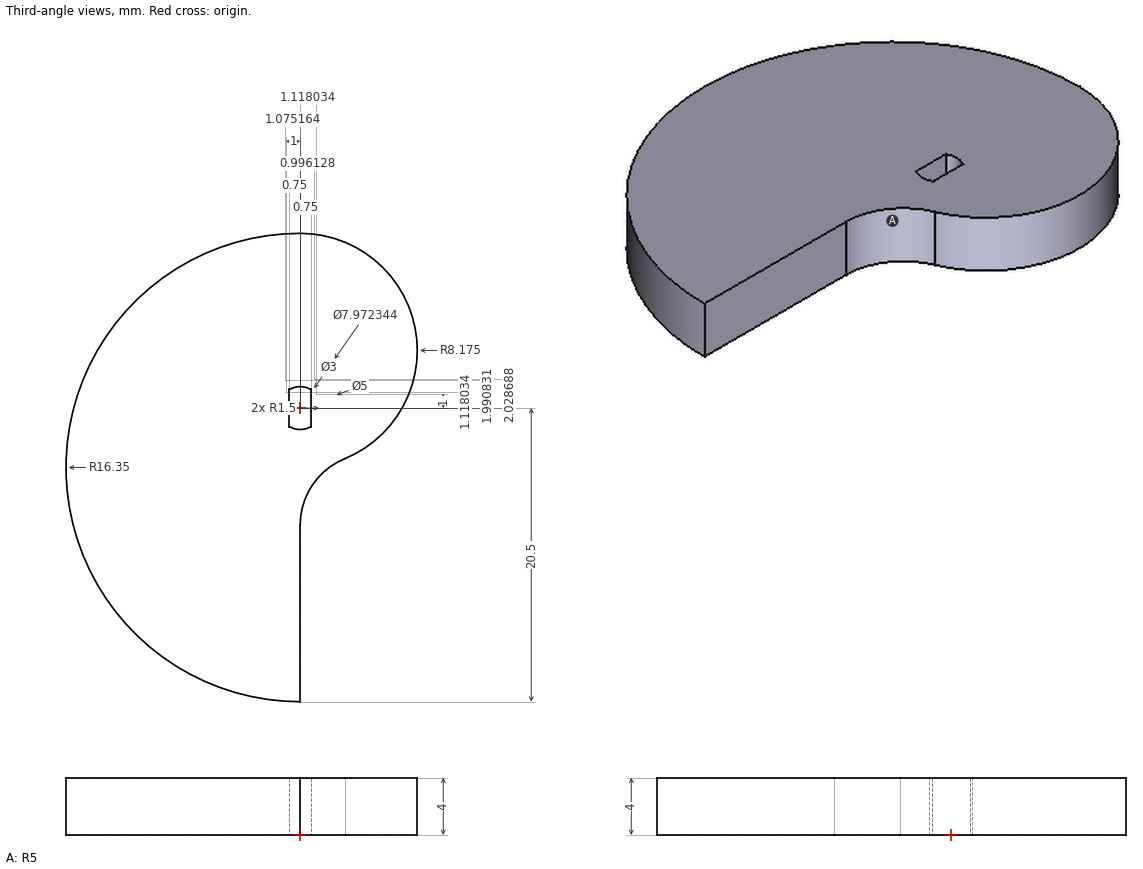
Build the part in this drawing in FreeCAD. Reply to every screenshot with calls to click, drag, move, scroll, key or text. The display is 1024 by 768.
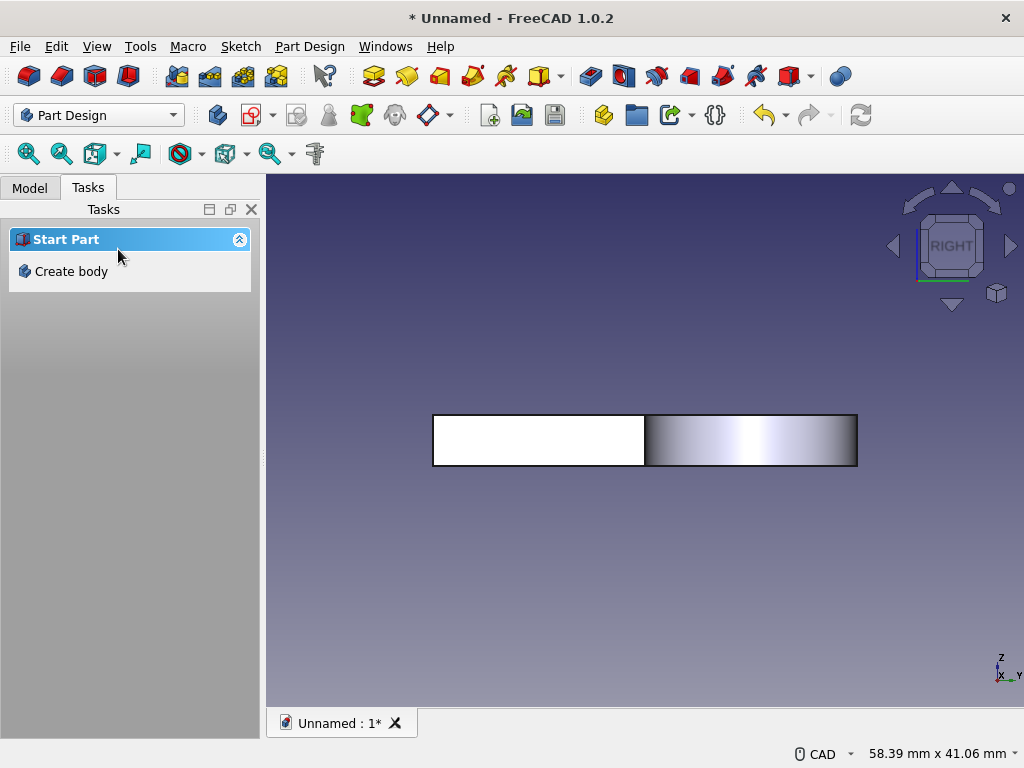
key(5)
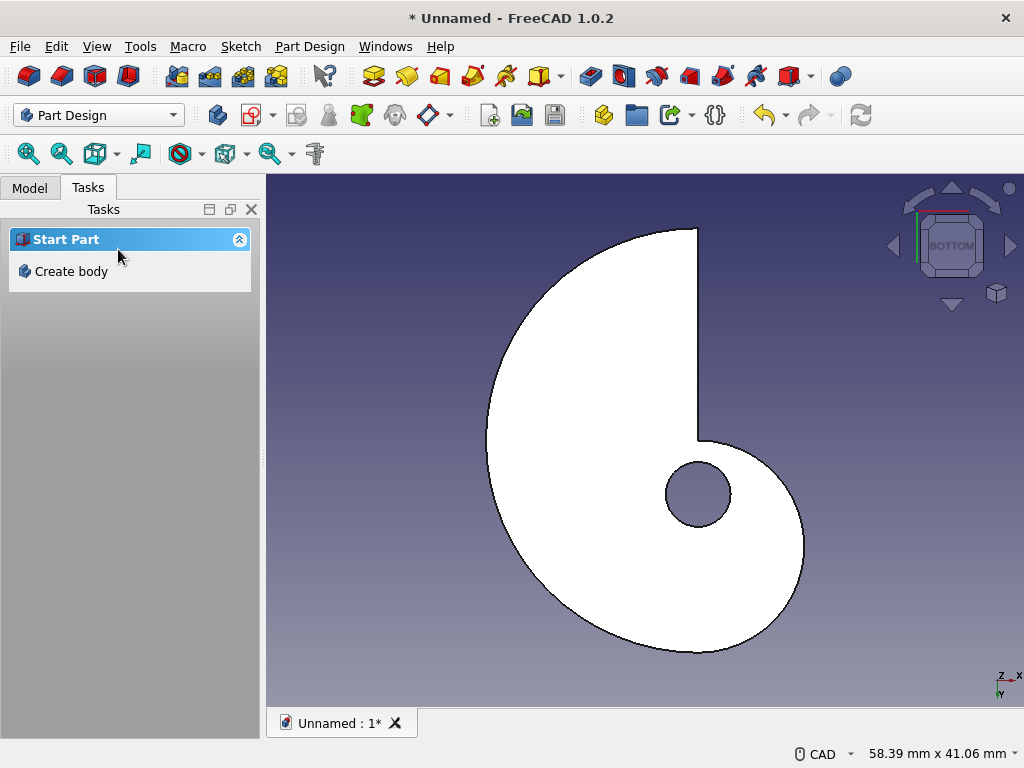
key(4)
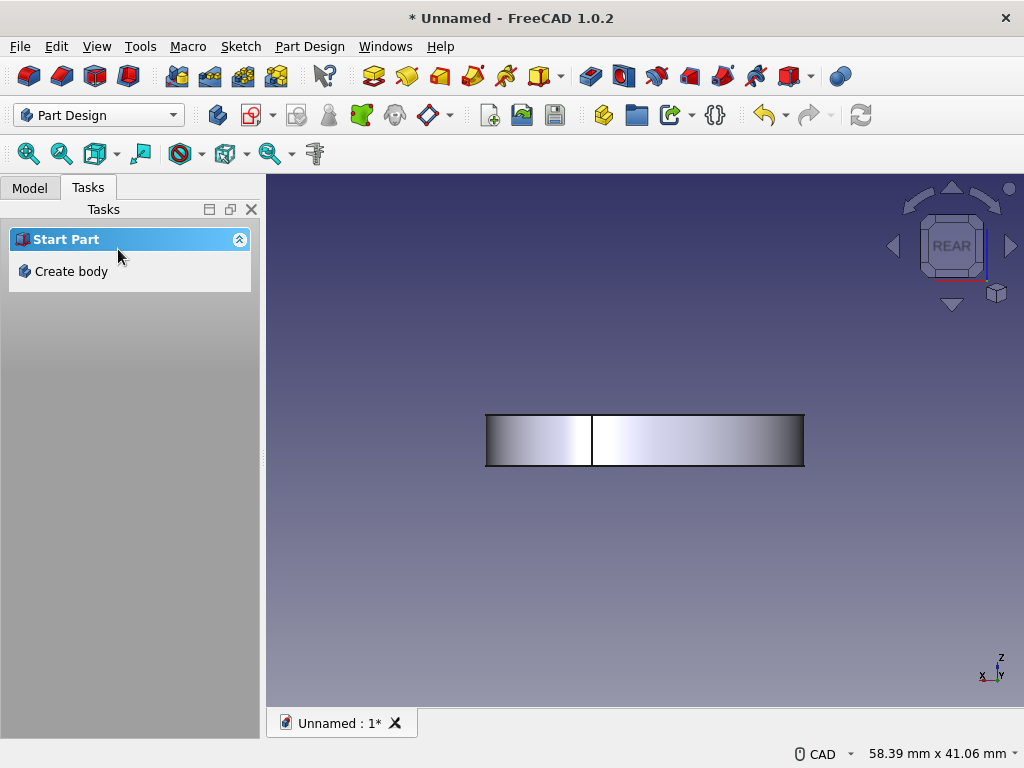
key(v)
key(f)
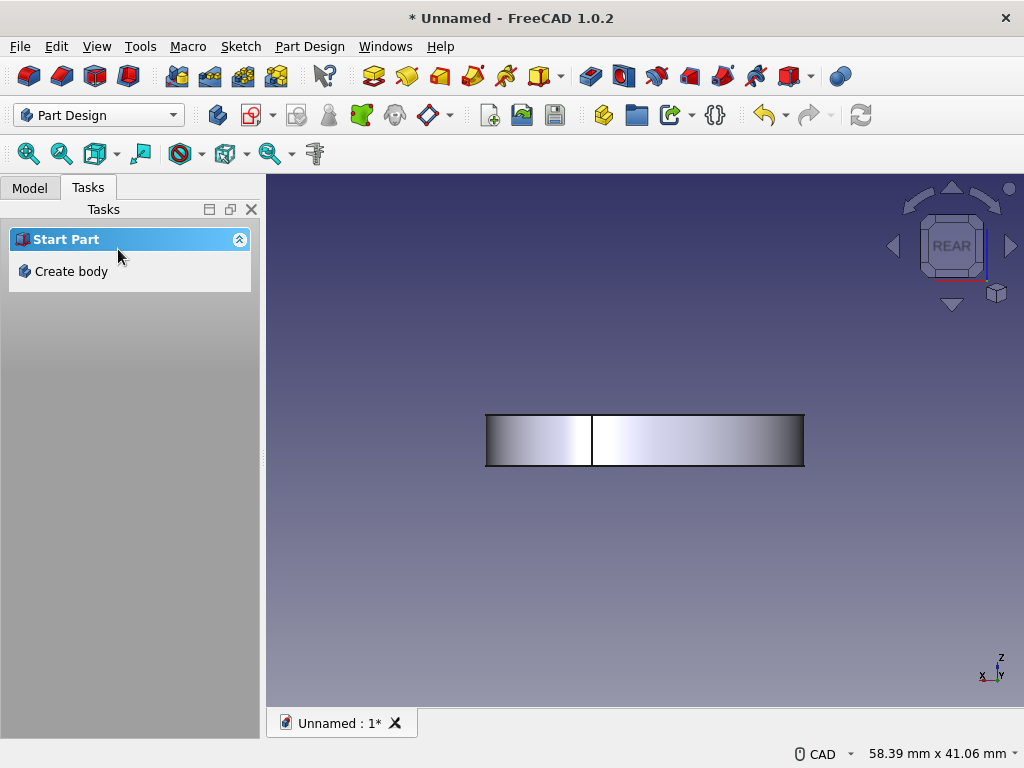
key(6)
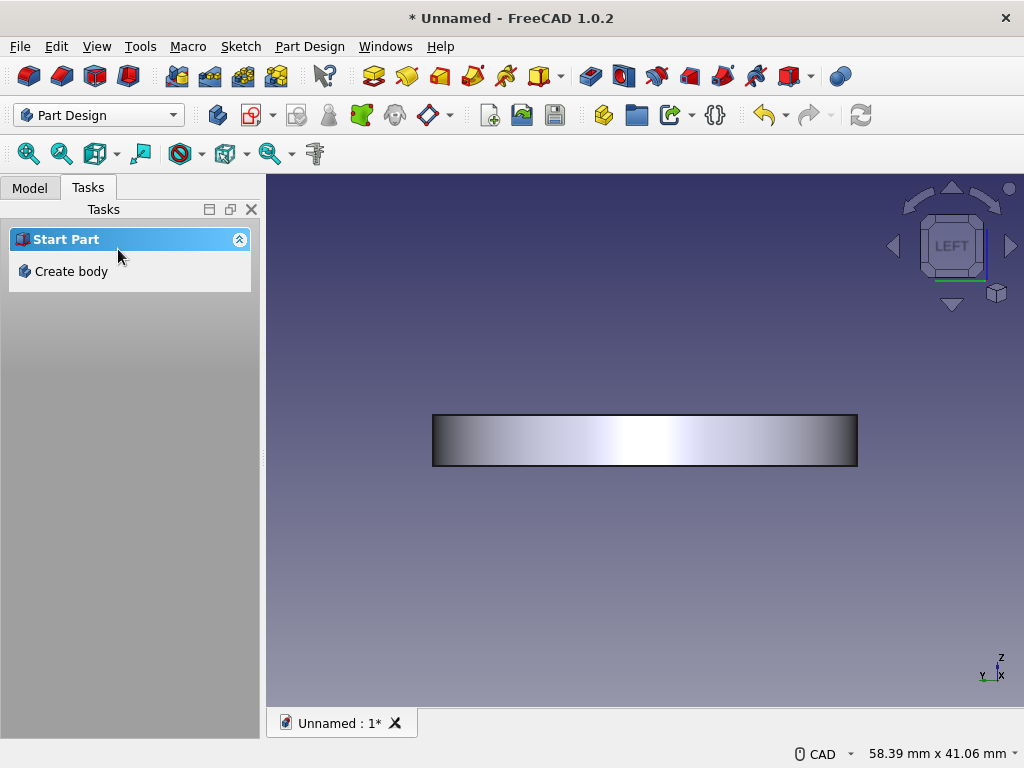
key(v)
key(3)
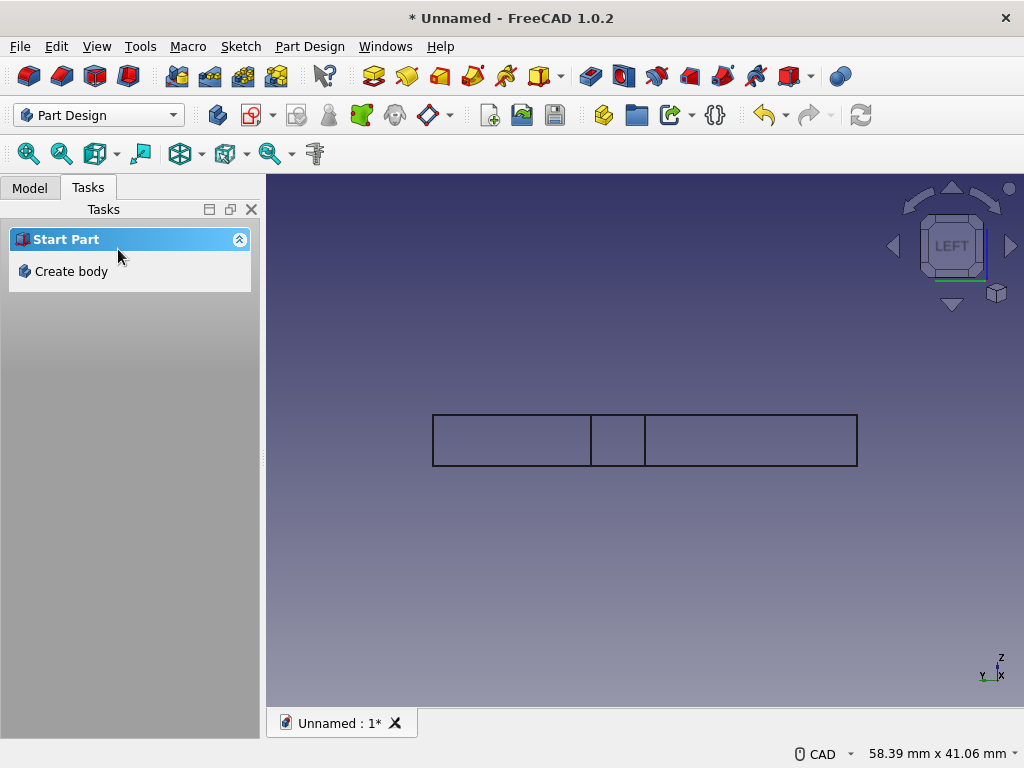
key(0)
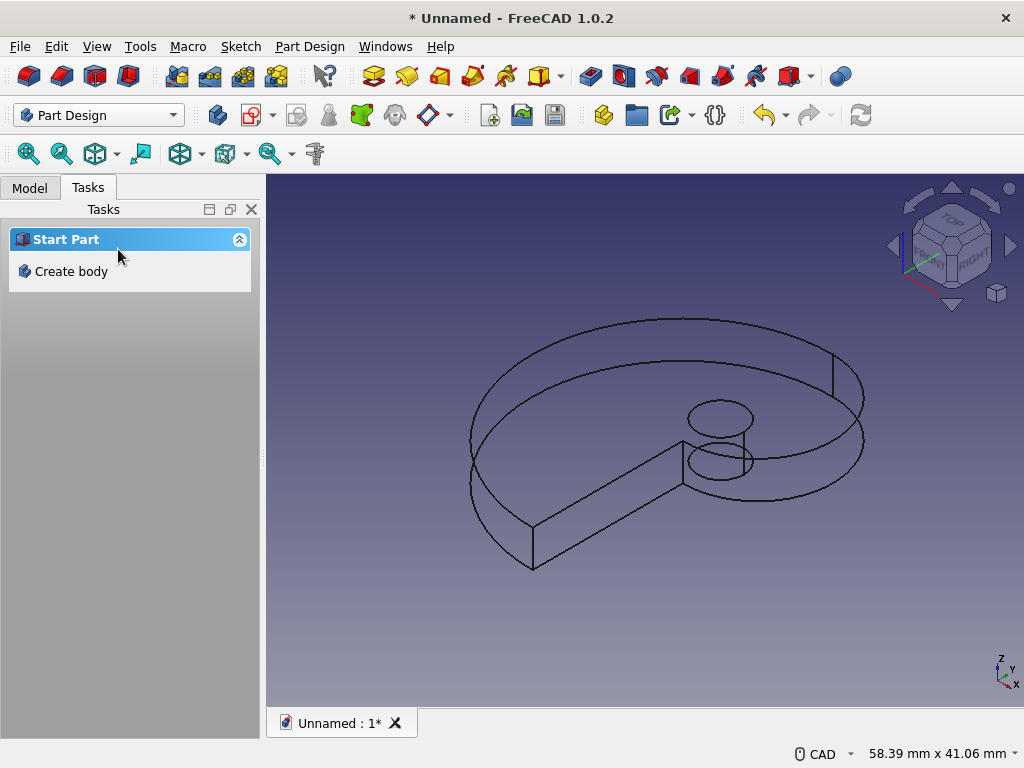
click(683, 461)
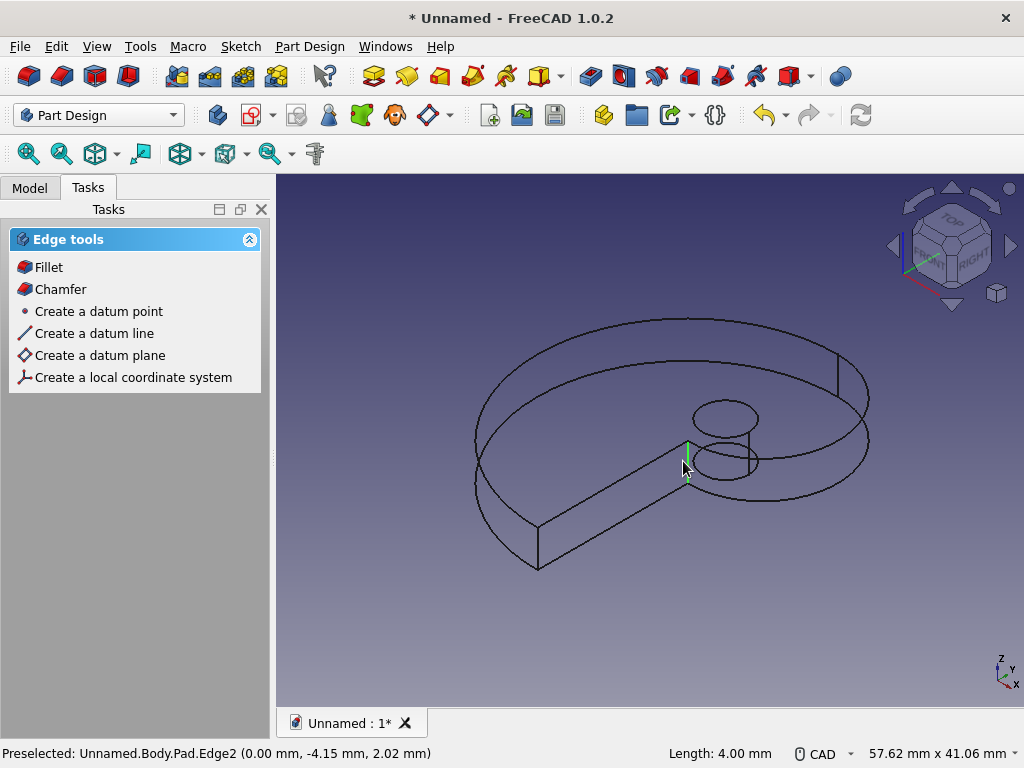
key(v)
key(1)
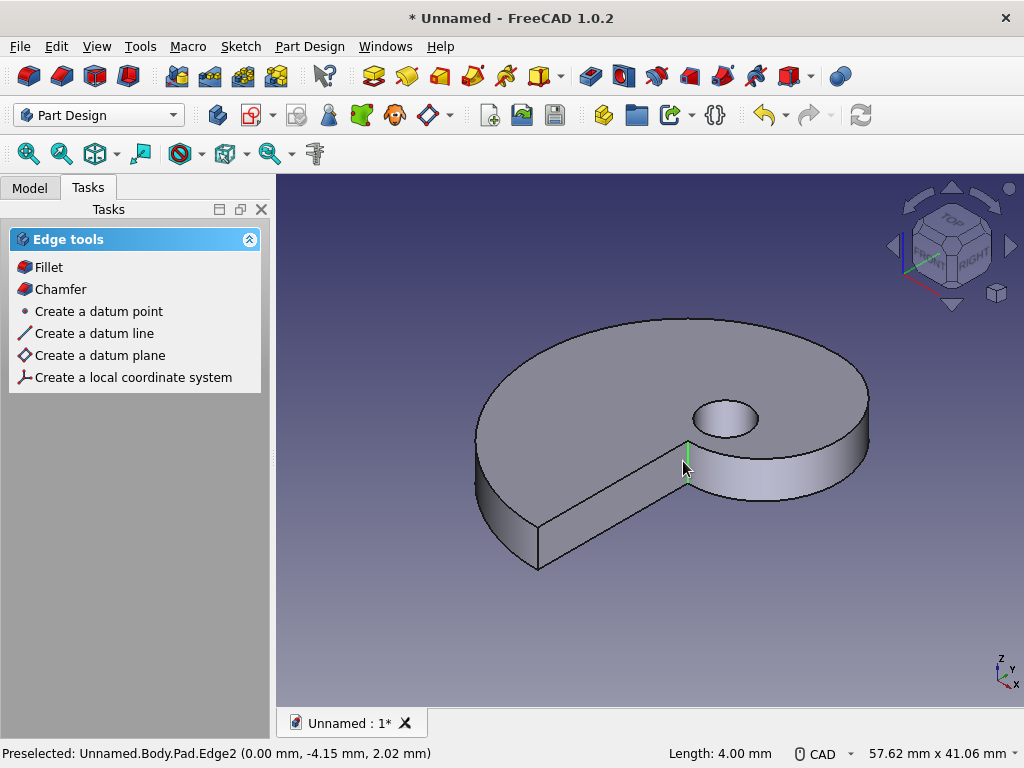
click(29, 76)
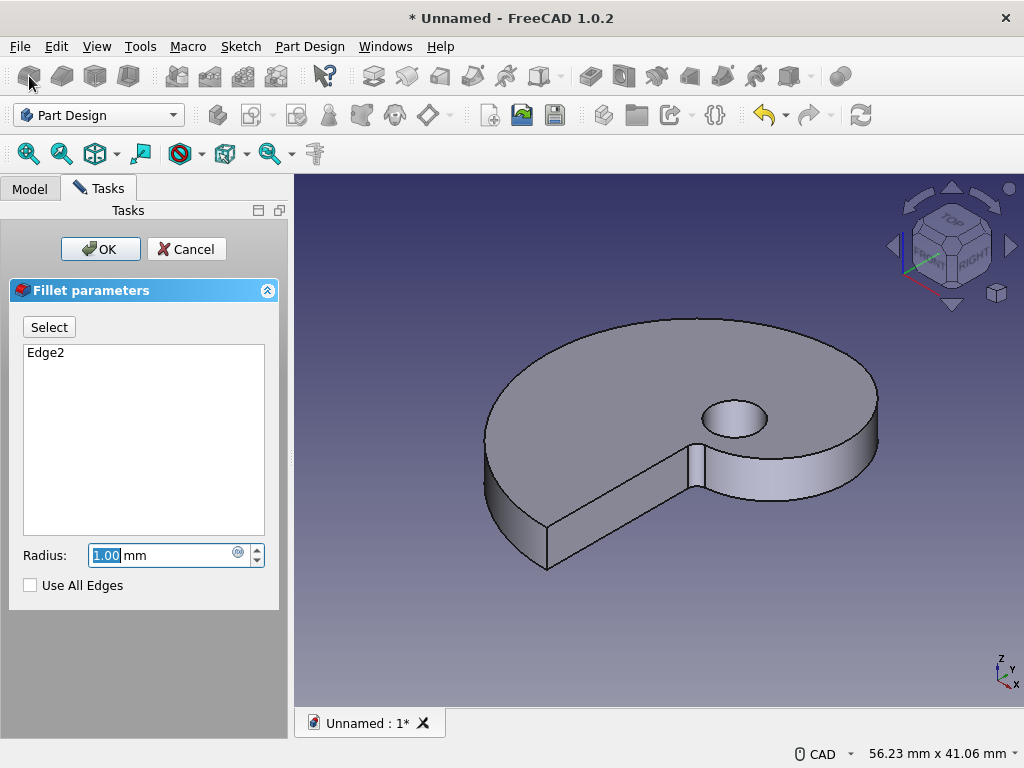
text(5)
key(Tab)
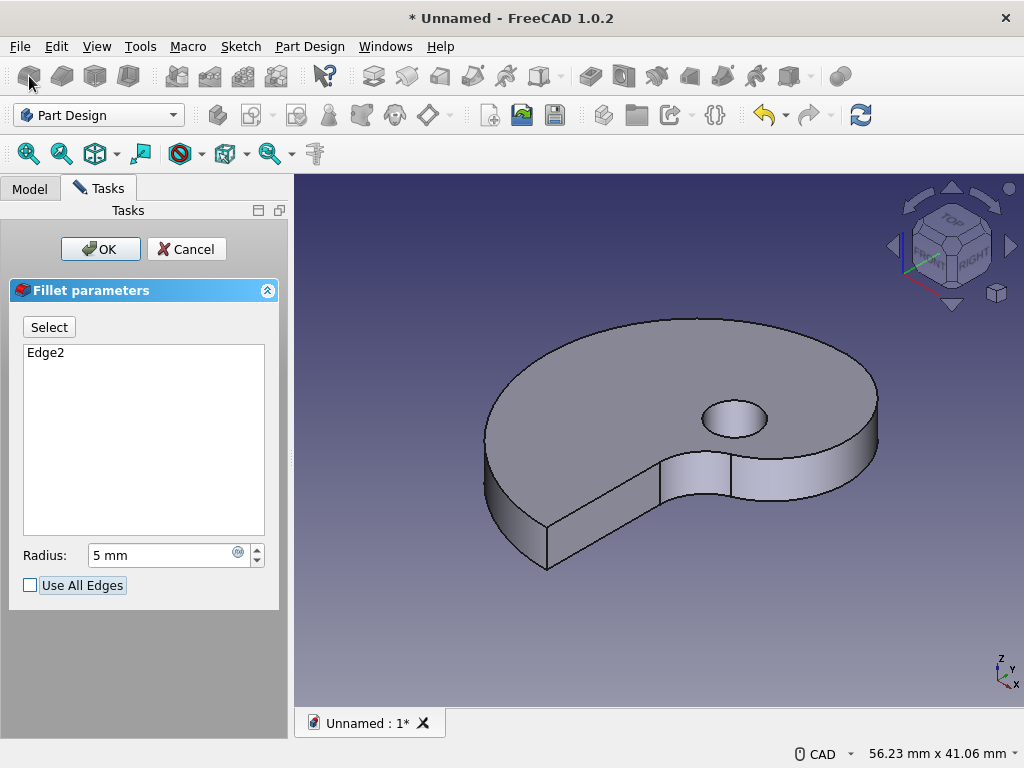
click(101, 249)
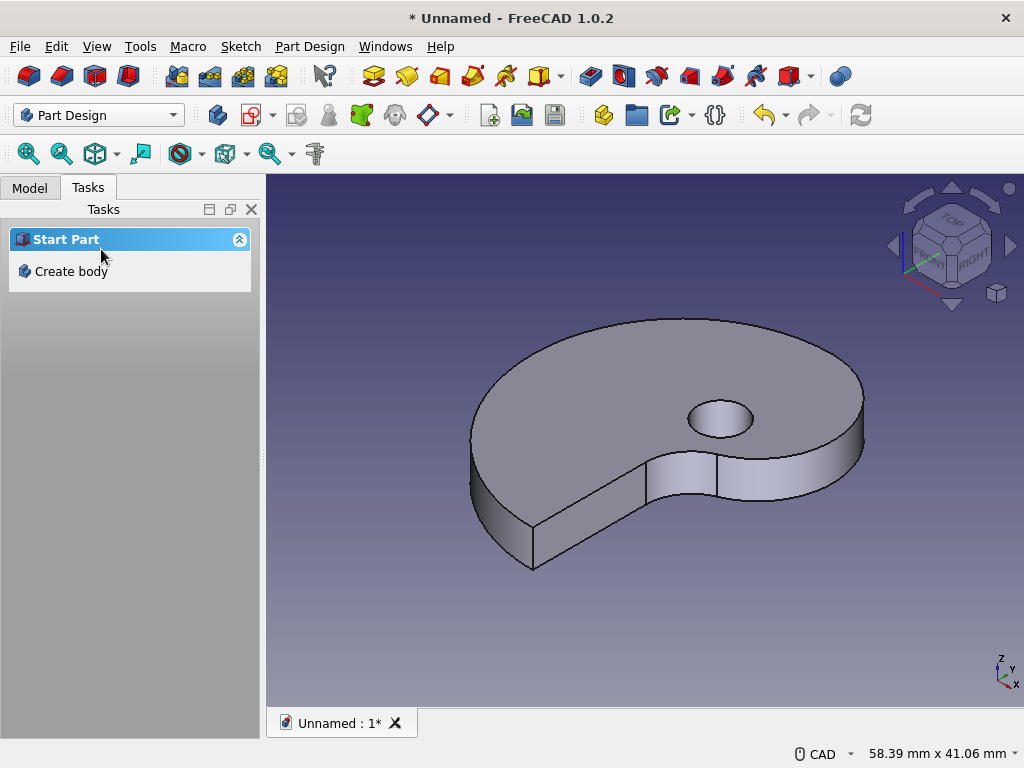
click(570, 425)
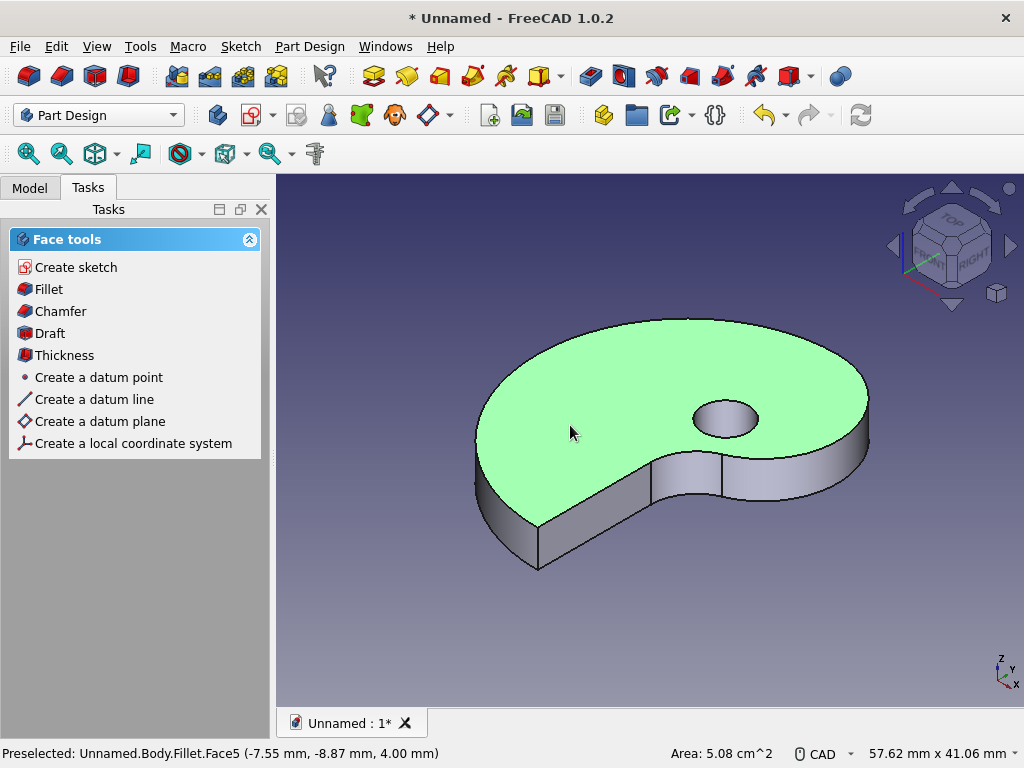
click(250, 116)